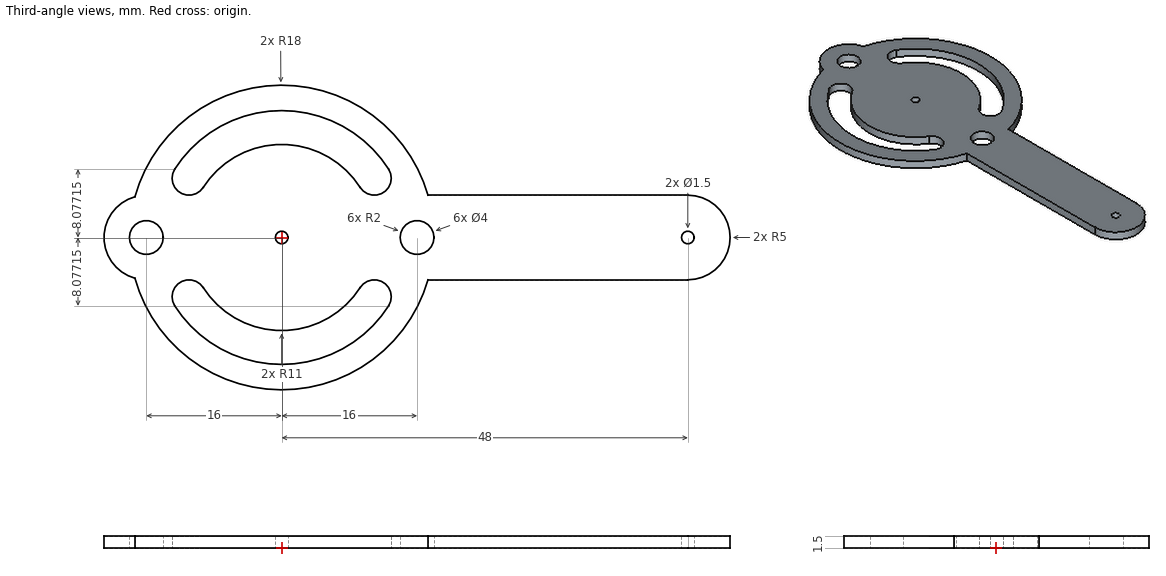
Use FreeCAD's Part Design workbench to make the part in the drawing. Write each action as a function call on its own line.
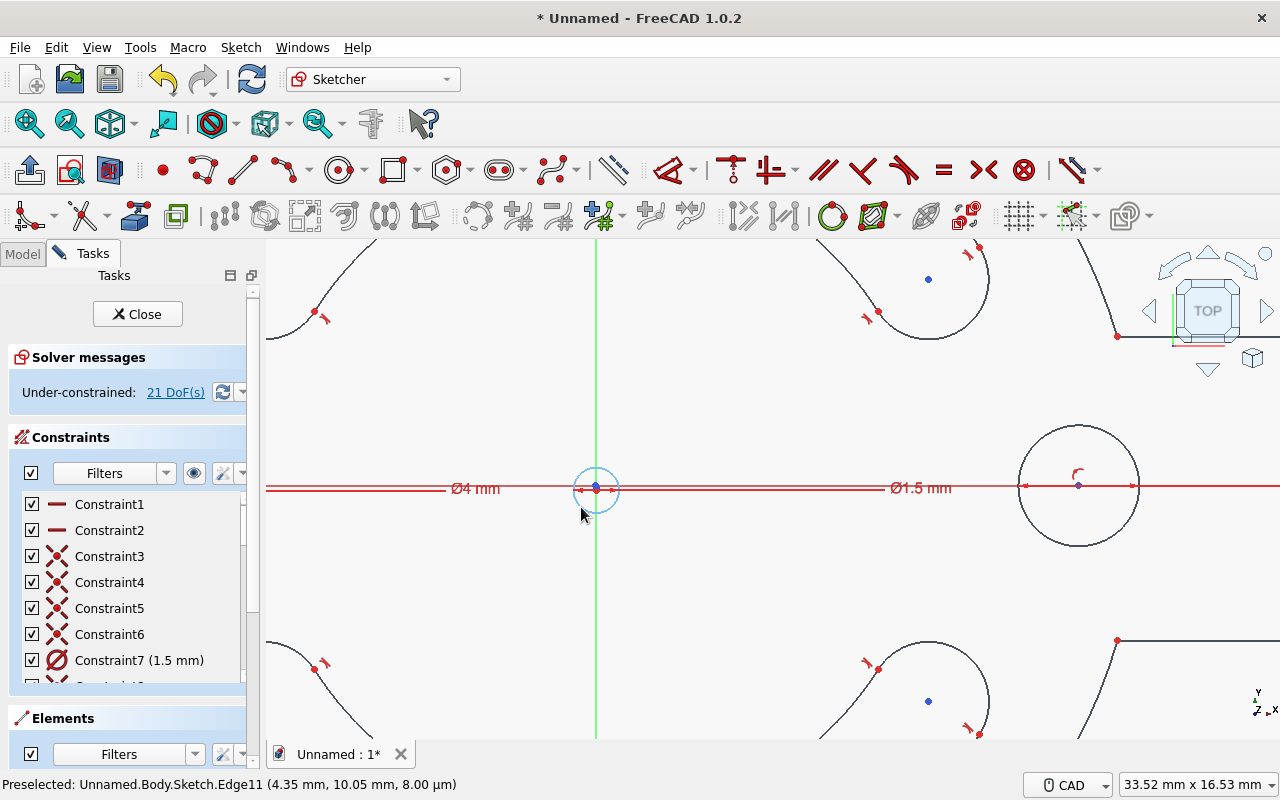
click(580, 506)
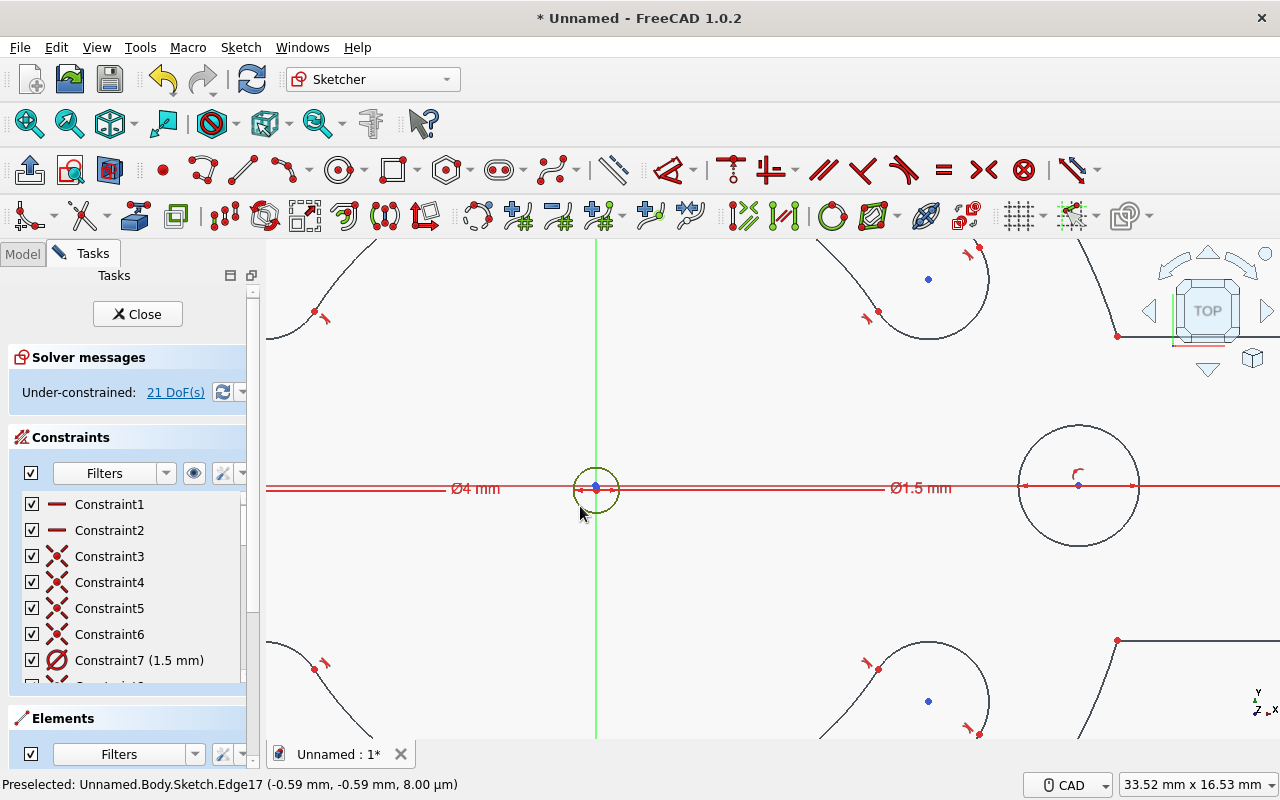
scroll(582, 490, down, 7)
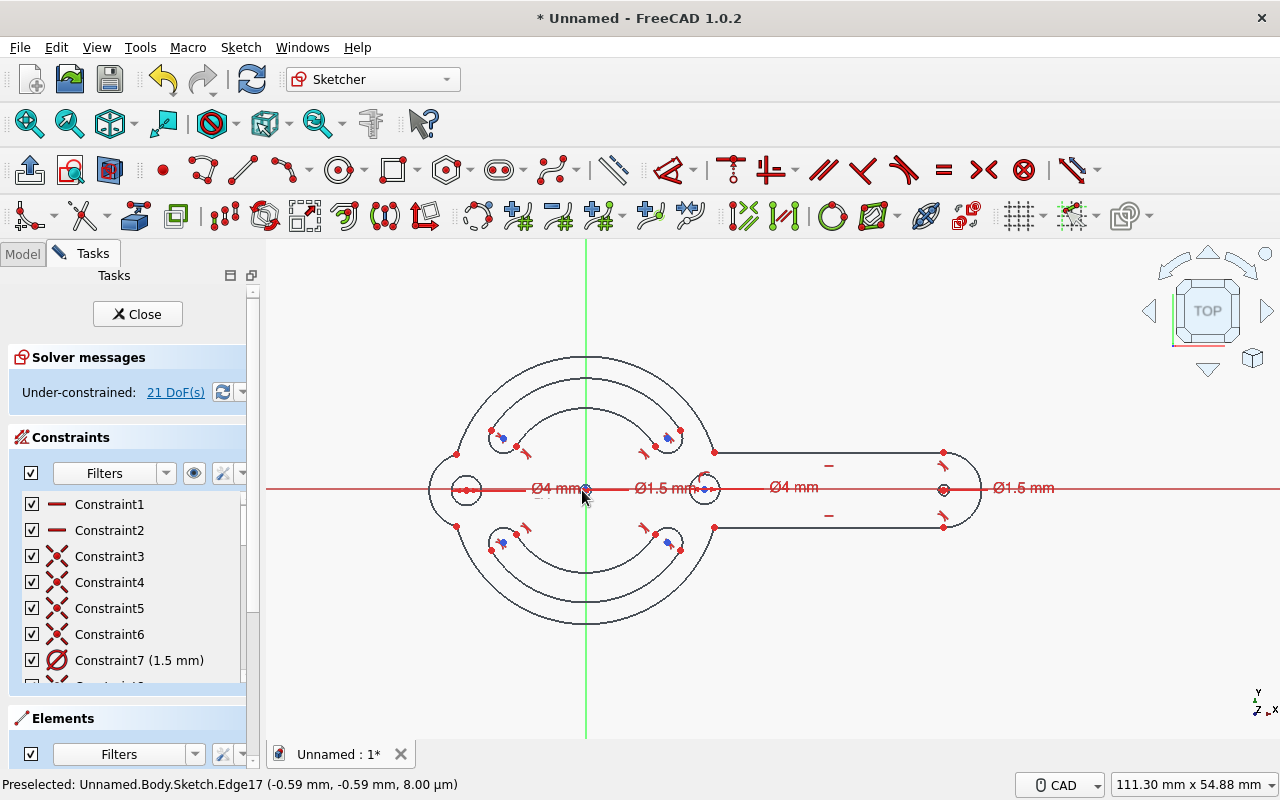
click(630, 387)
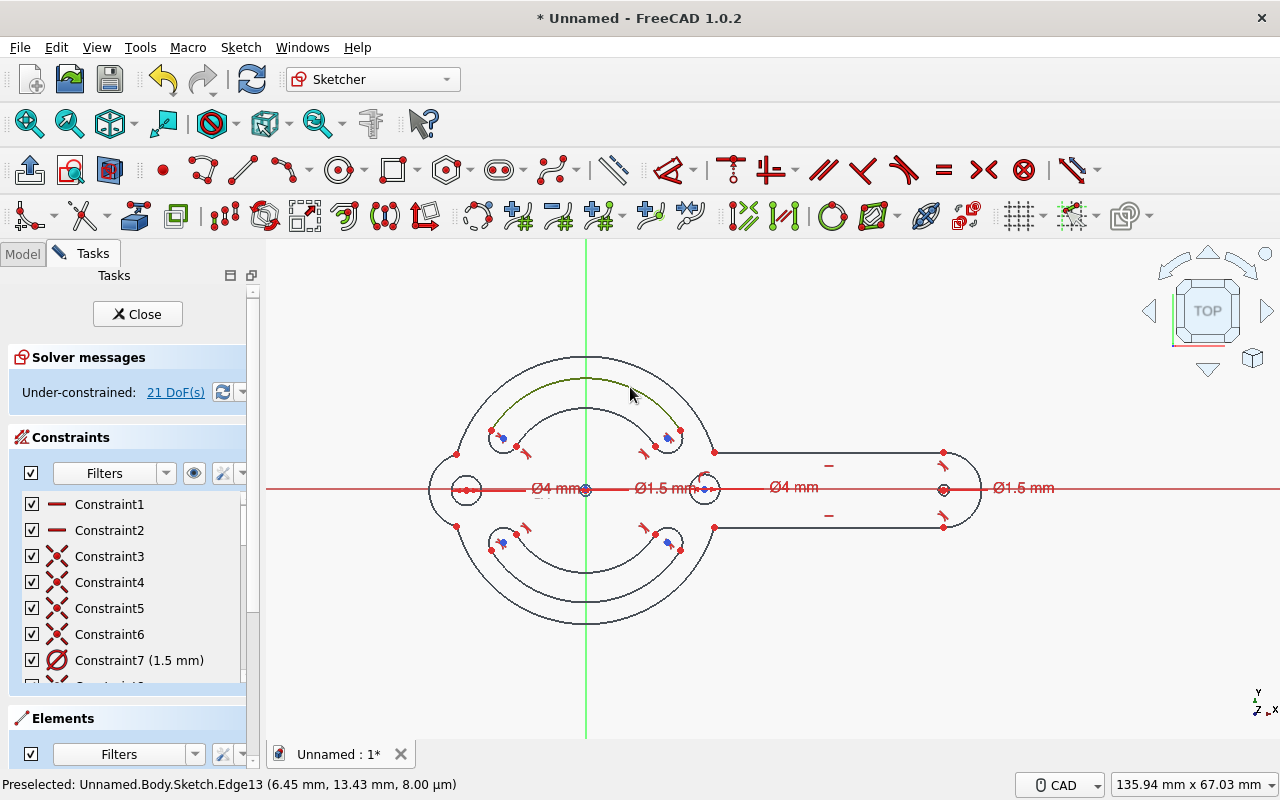
click(732, 170)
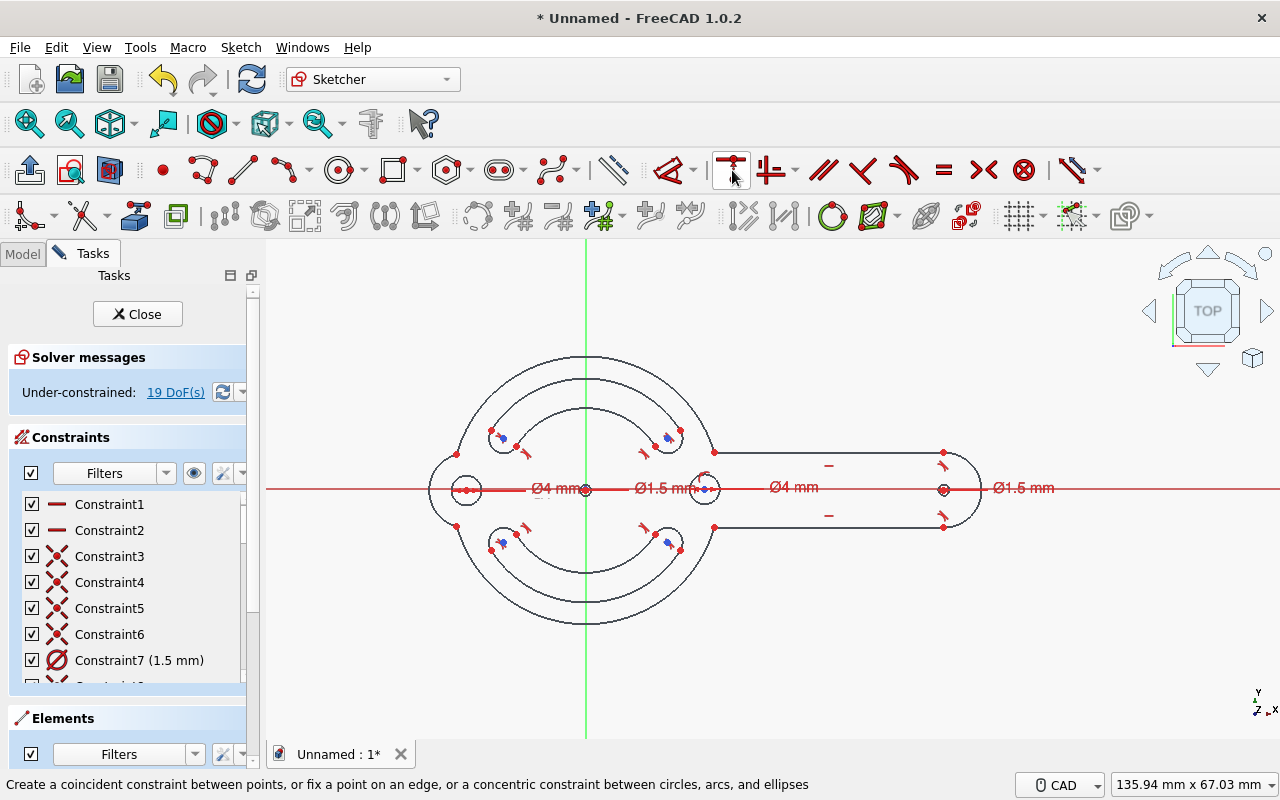
scroll(586, 490, up, 10)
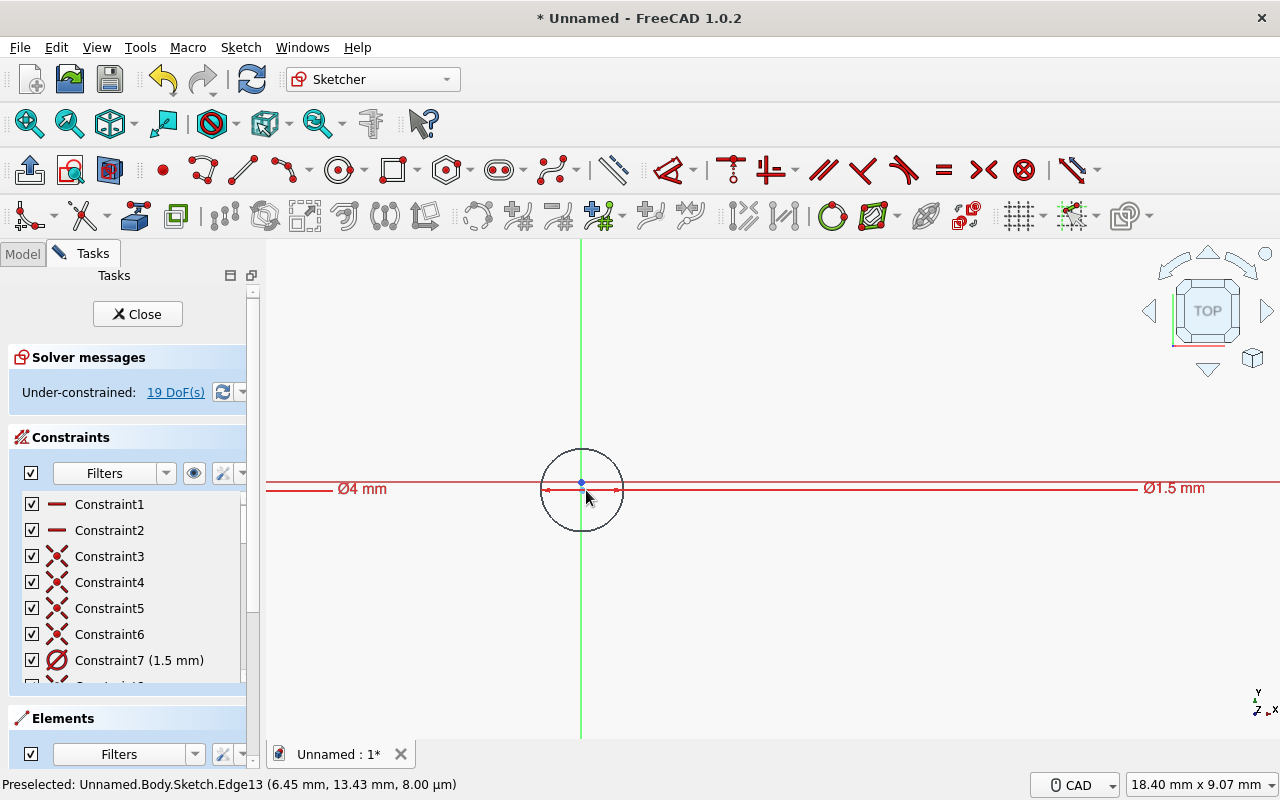
drag(571, 472, 592, 500)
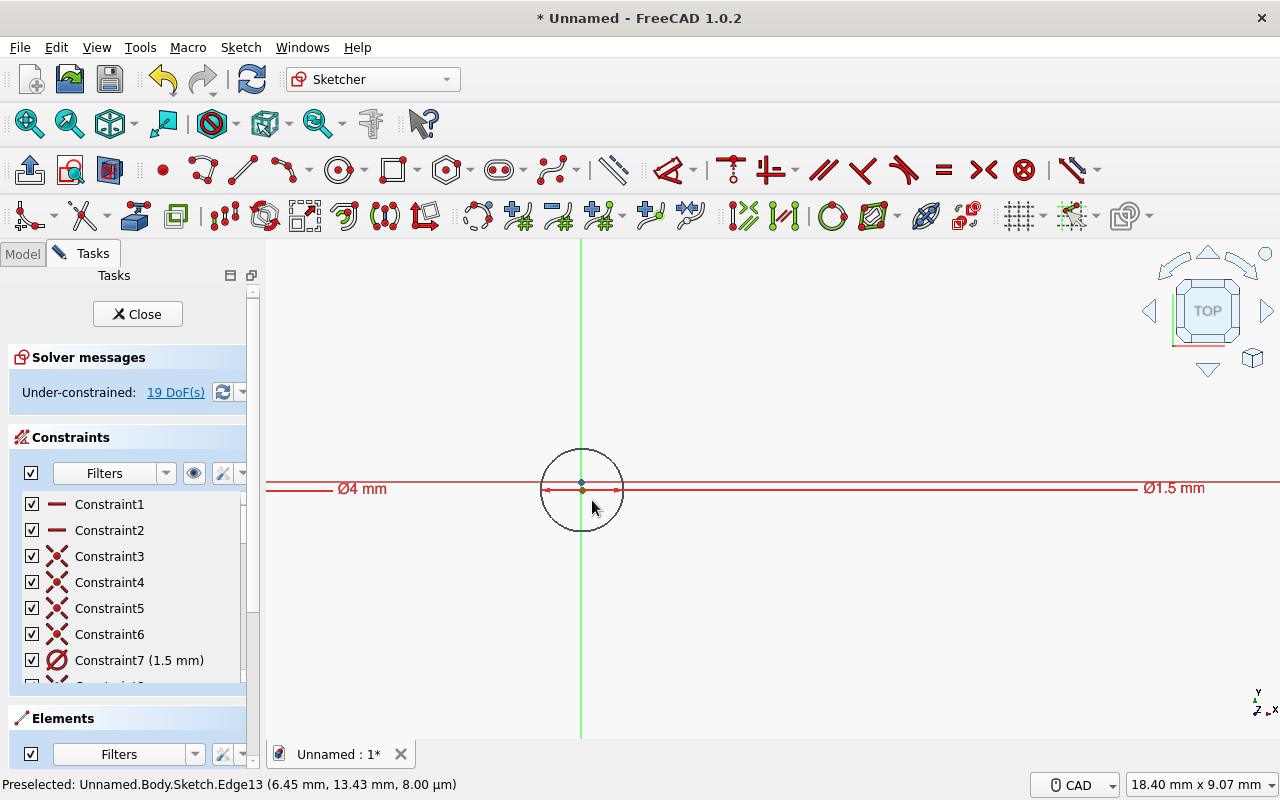
click(732, 170)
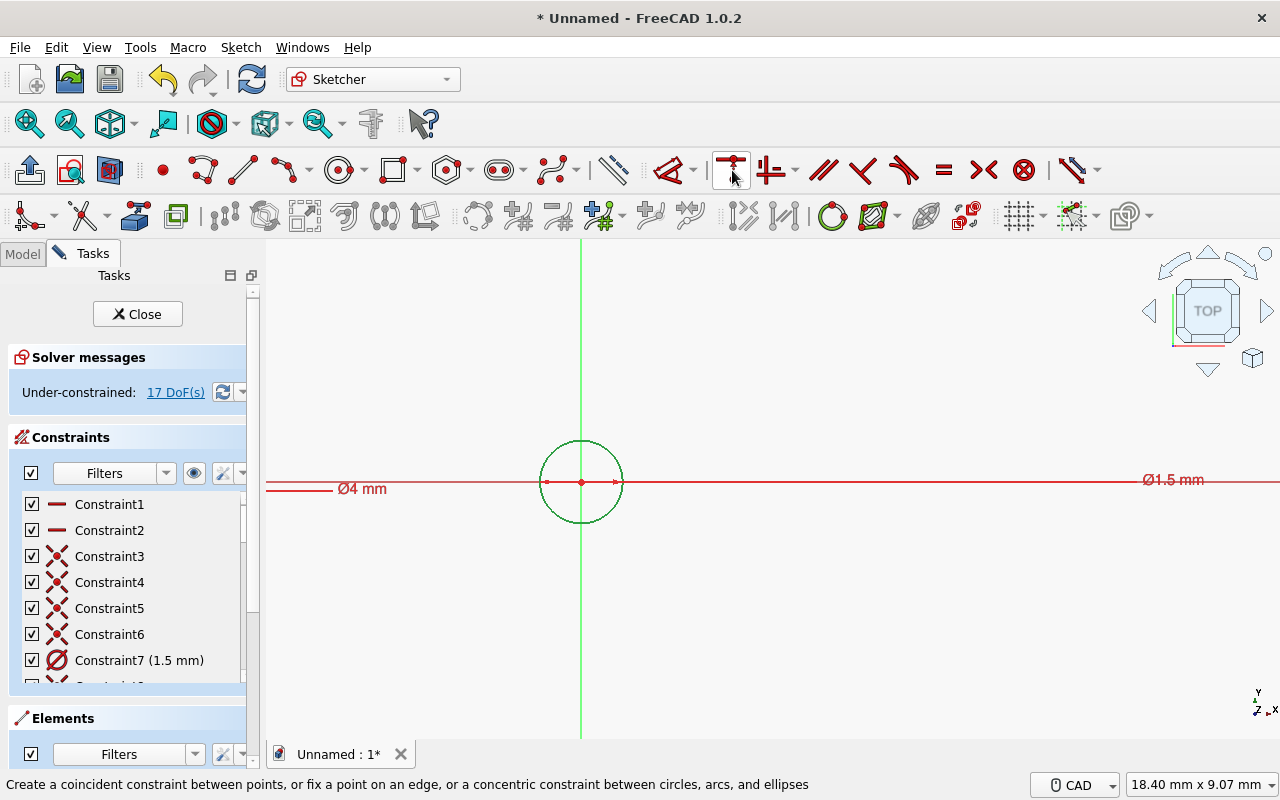
scroll(586, 490, down, 10)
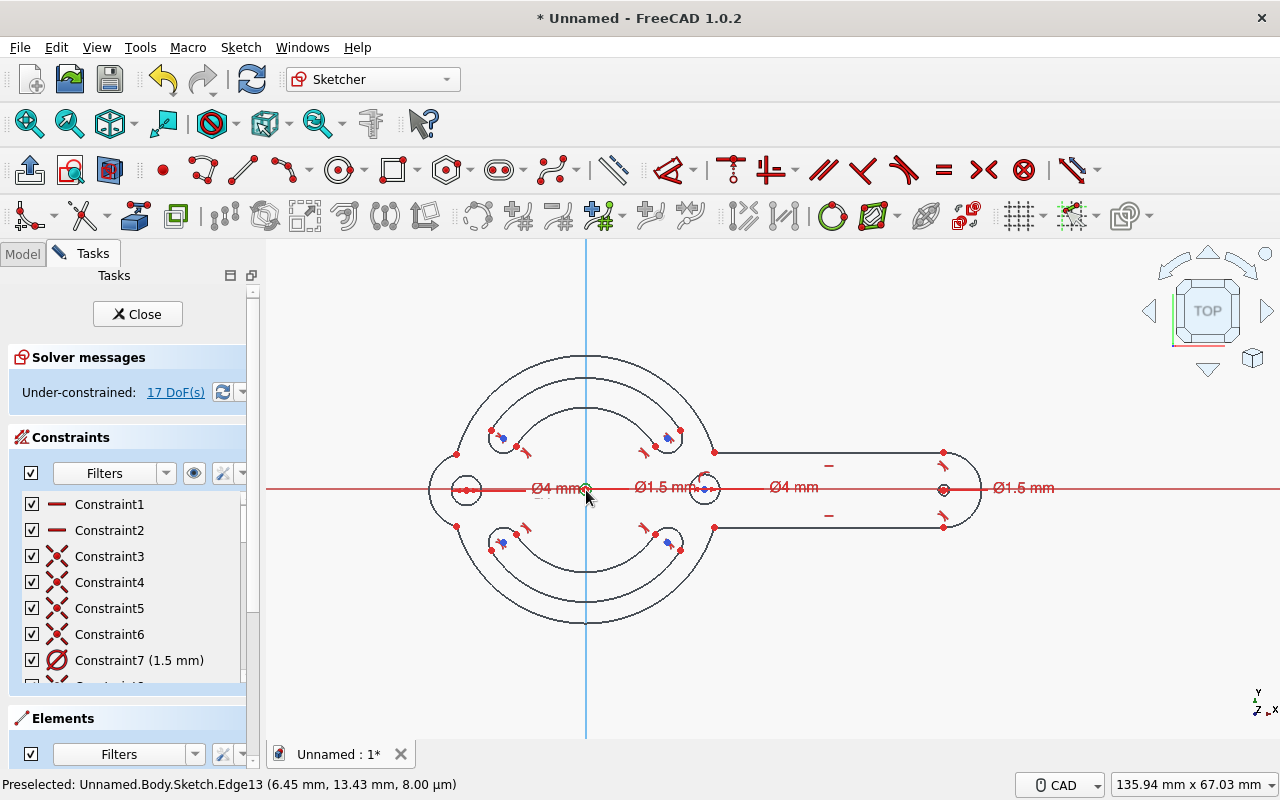
click(974, 512)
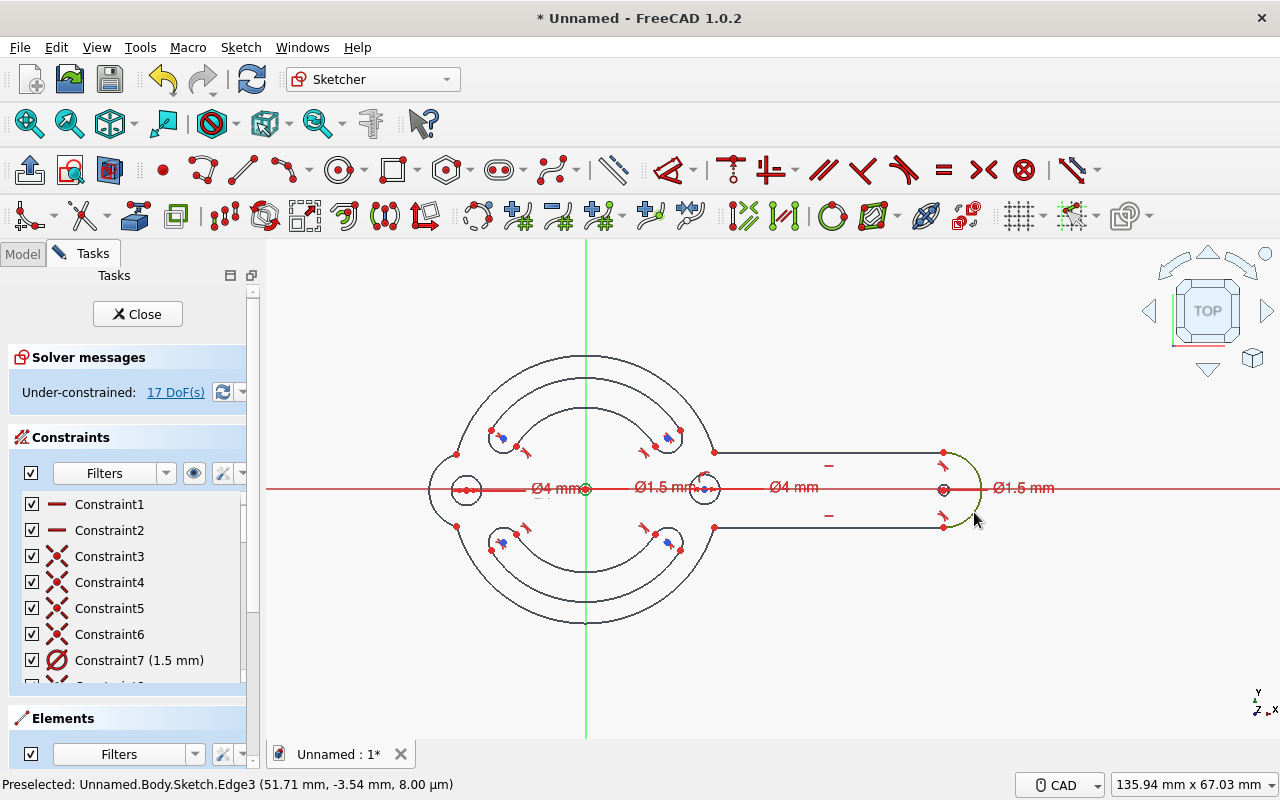
click(434, 472)